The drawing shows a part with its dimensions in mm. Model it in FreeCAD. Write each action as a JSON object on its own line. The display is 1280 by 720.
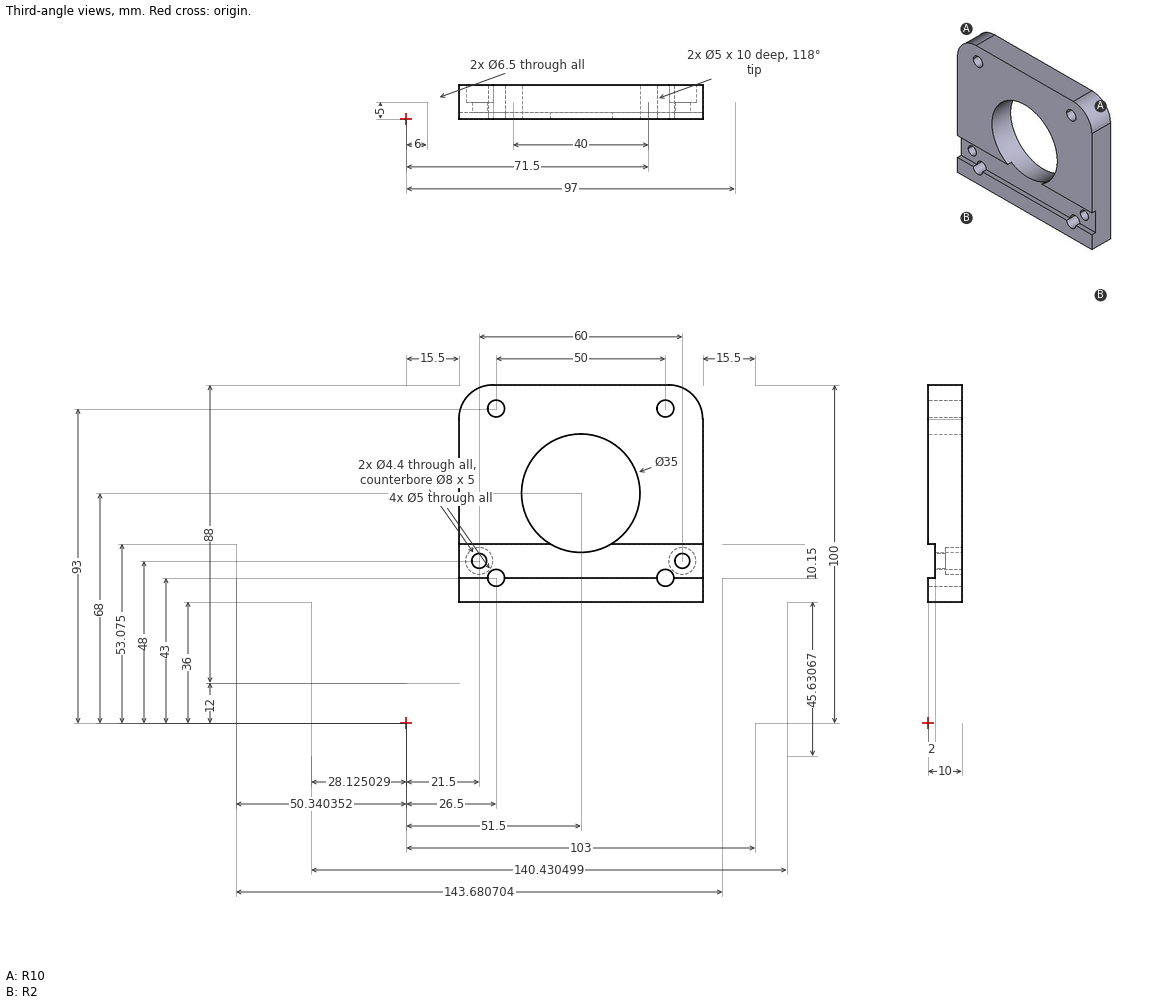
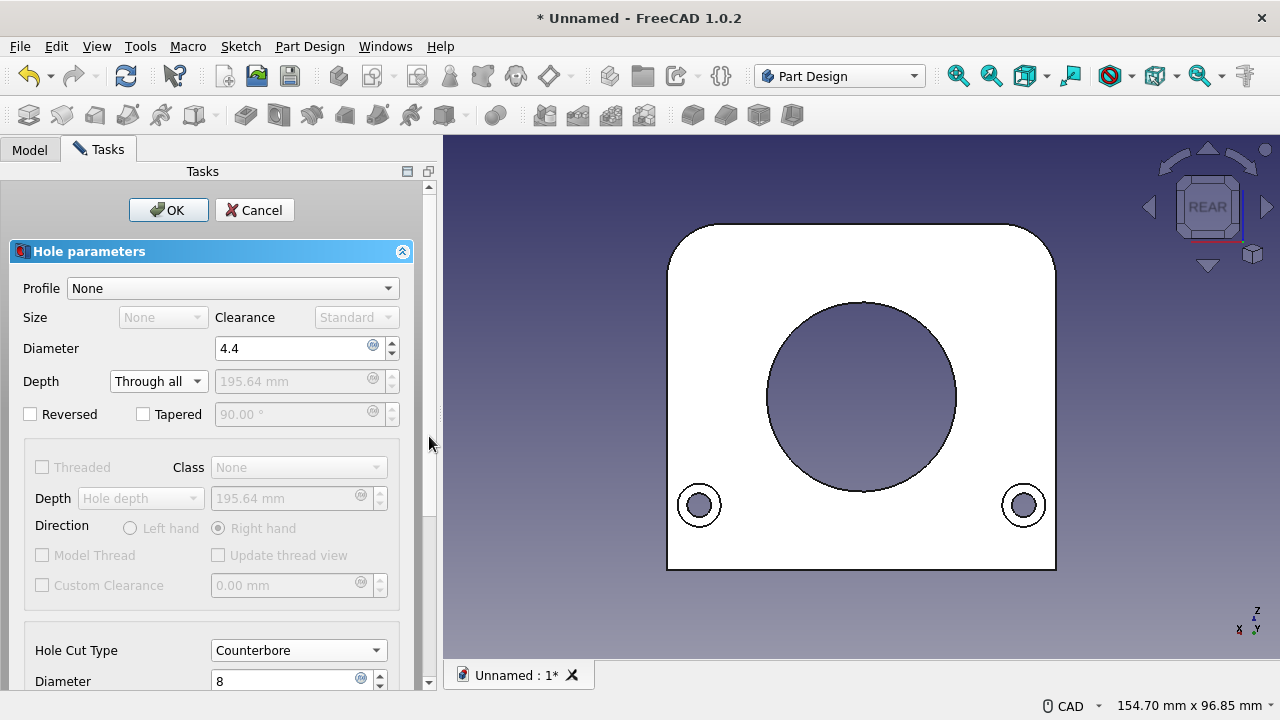
{"action": "left_click", "coordinate": [169, 210]}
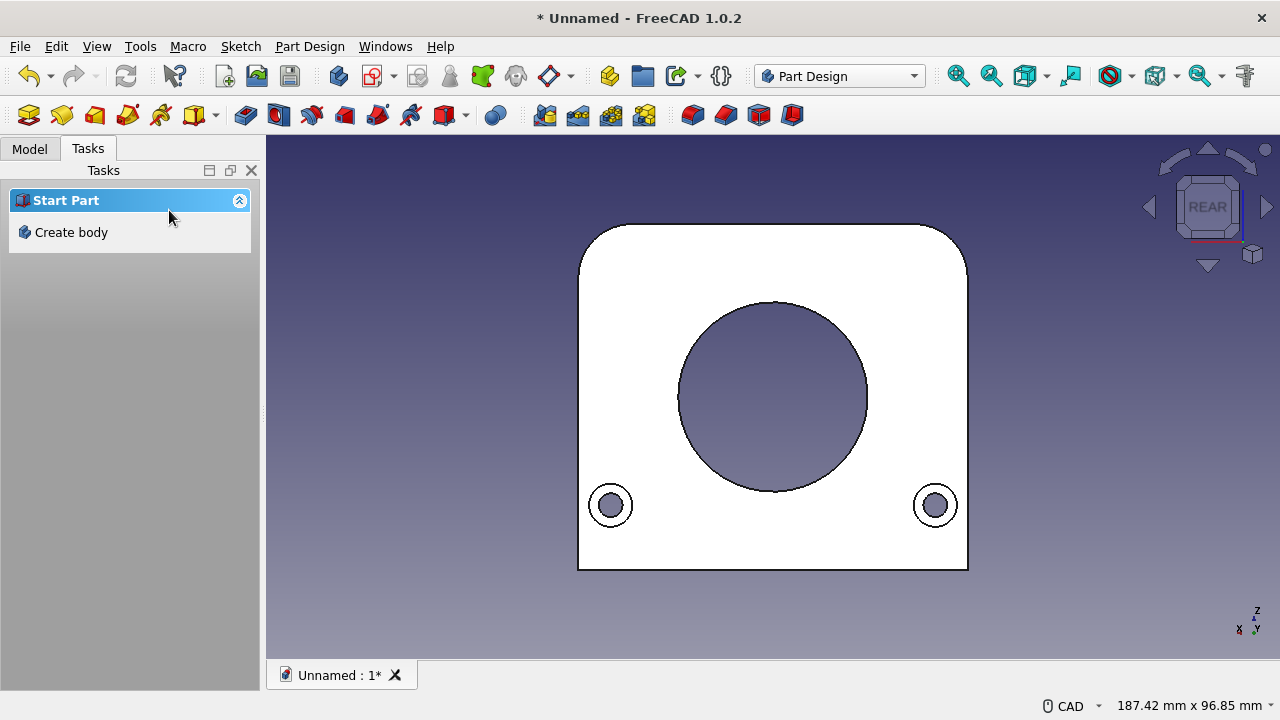
{"action": "left_click", "coordinate": [662, 297]}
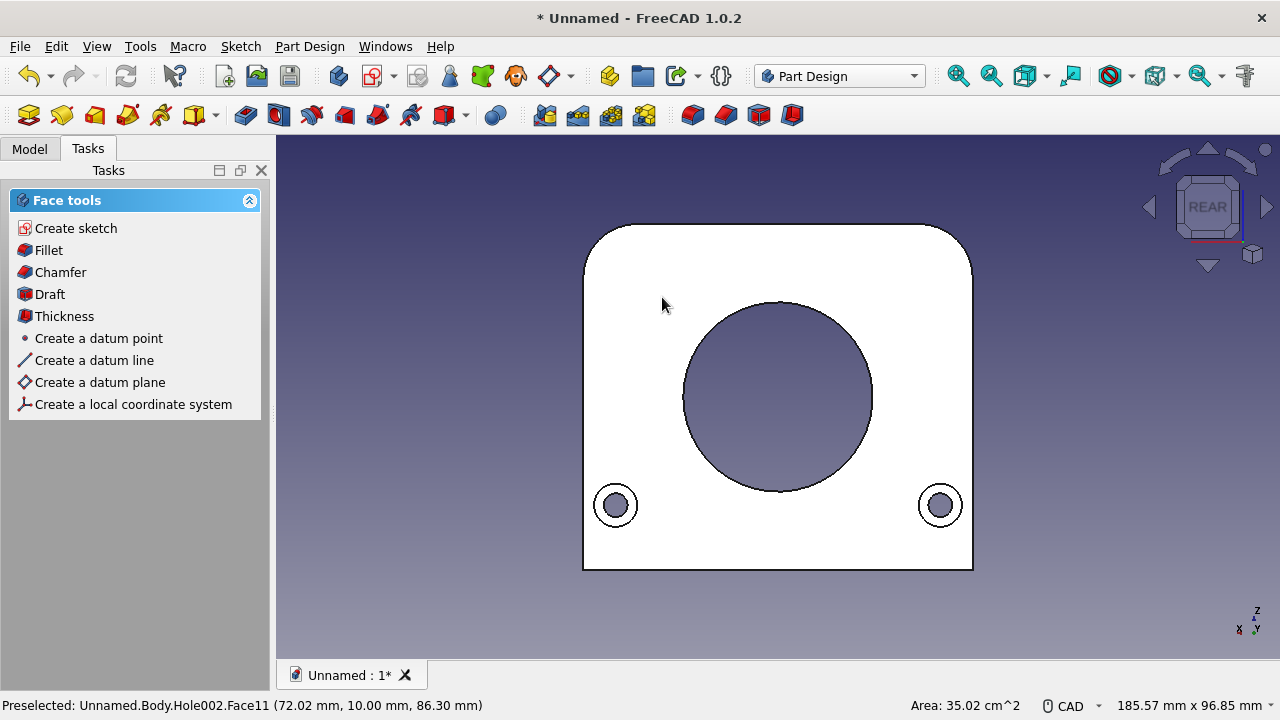
{"action": "left_click", "coordinate": [372, 76]}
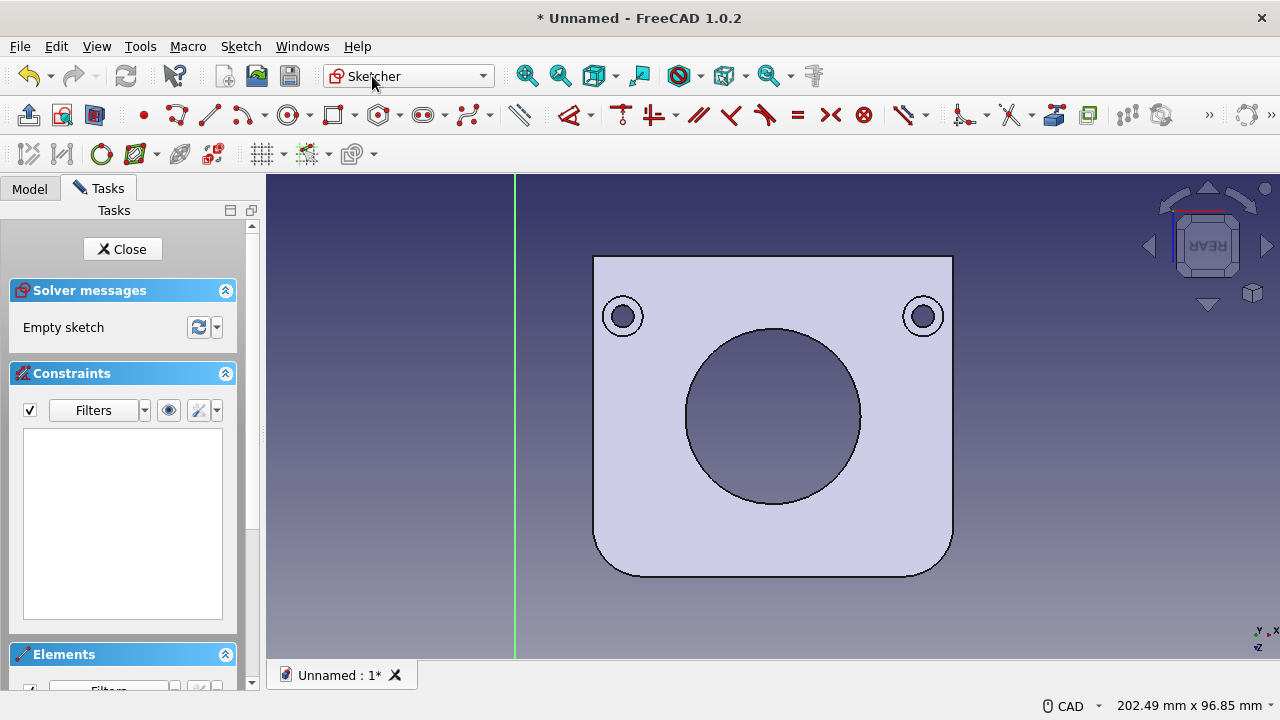
{"action": "scroll", "coordinate": [687, 623], "scroll_direction": "down", "scroll_amount": 2}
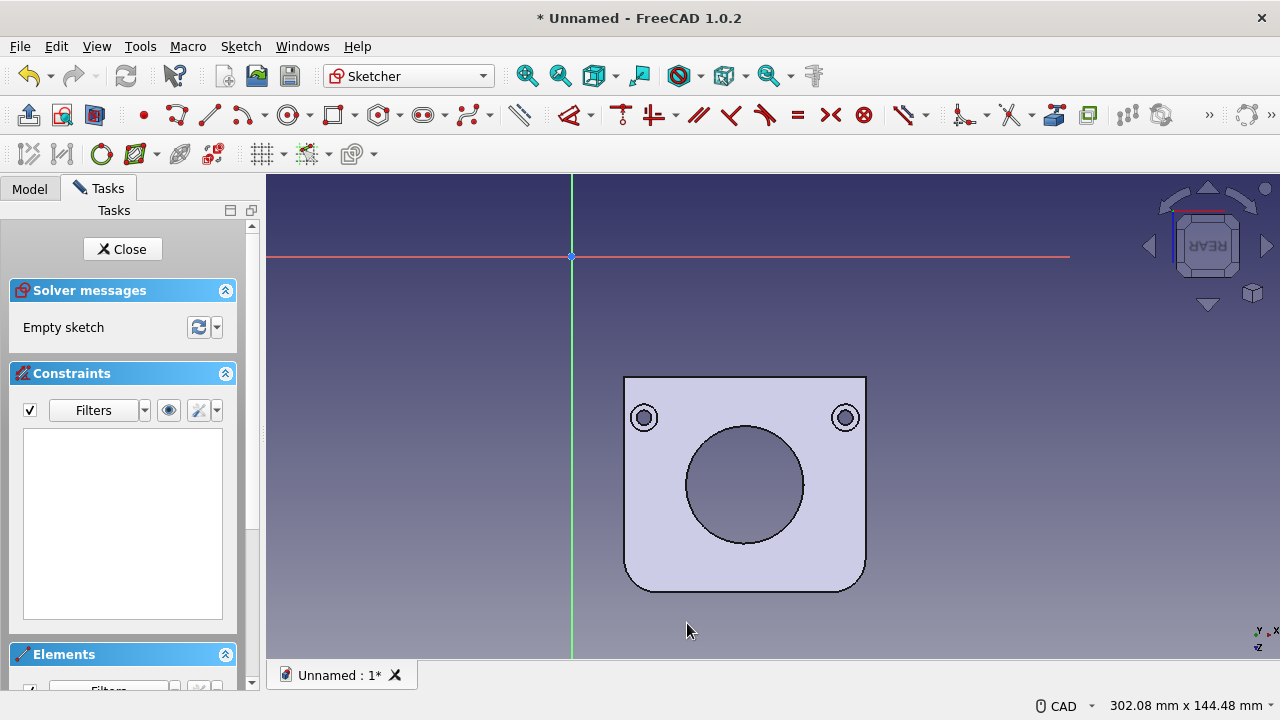
{"action": "left_click", "coordinate": [288, 116]}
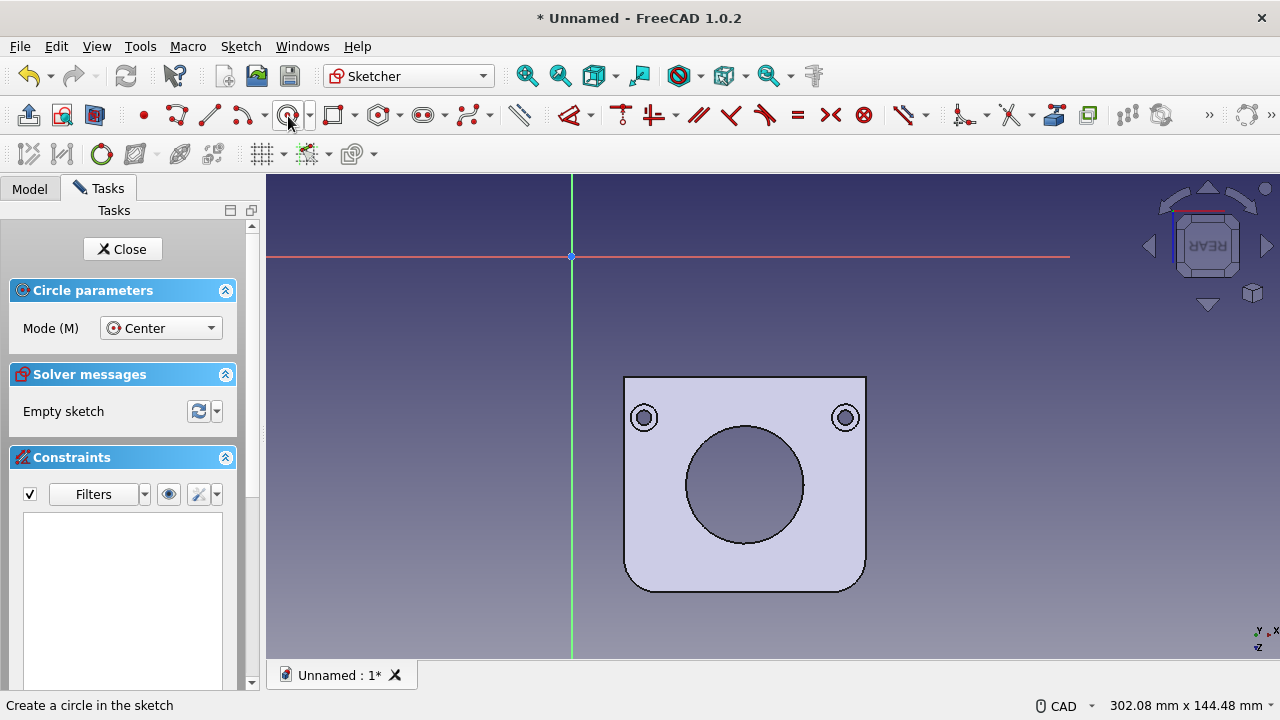
{"action": "scroll", "coordinate": [661, 401], "scroll_direction": "up", "scroll_amount": 5}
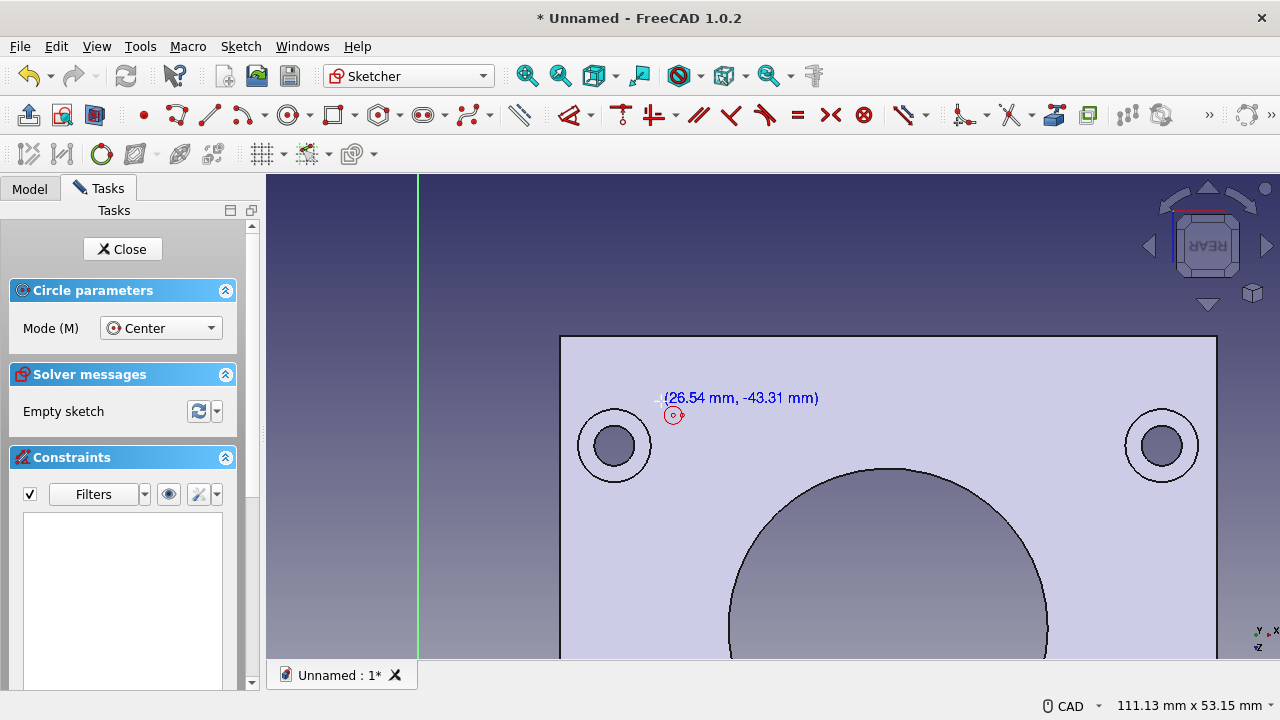
{"action": "left_click", "coordinate": [660, 400]}
{"action": "mouse_move", "coordinate": [676, 384]}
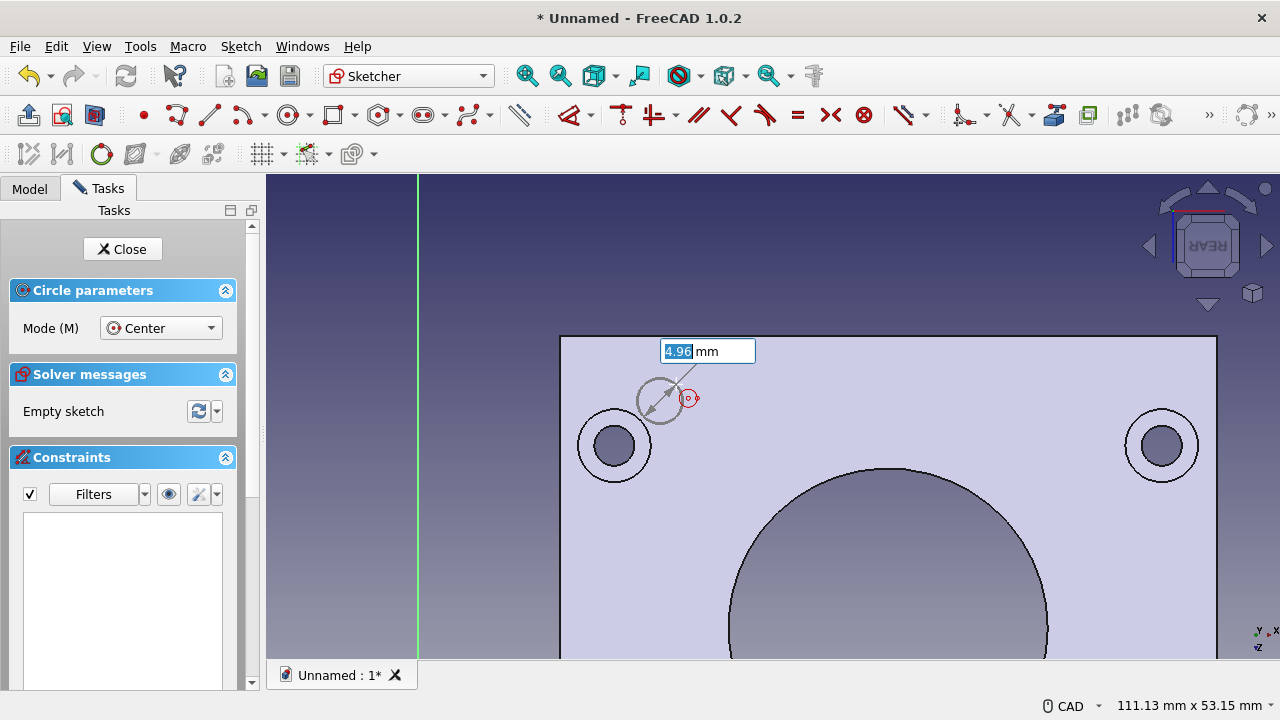
{"action": "type", "text": "5"}
{"action": "key", "text": "Return"}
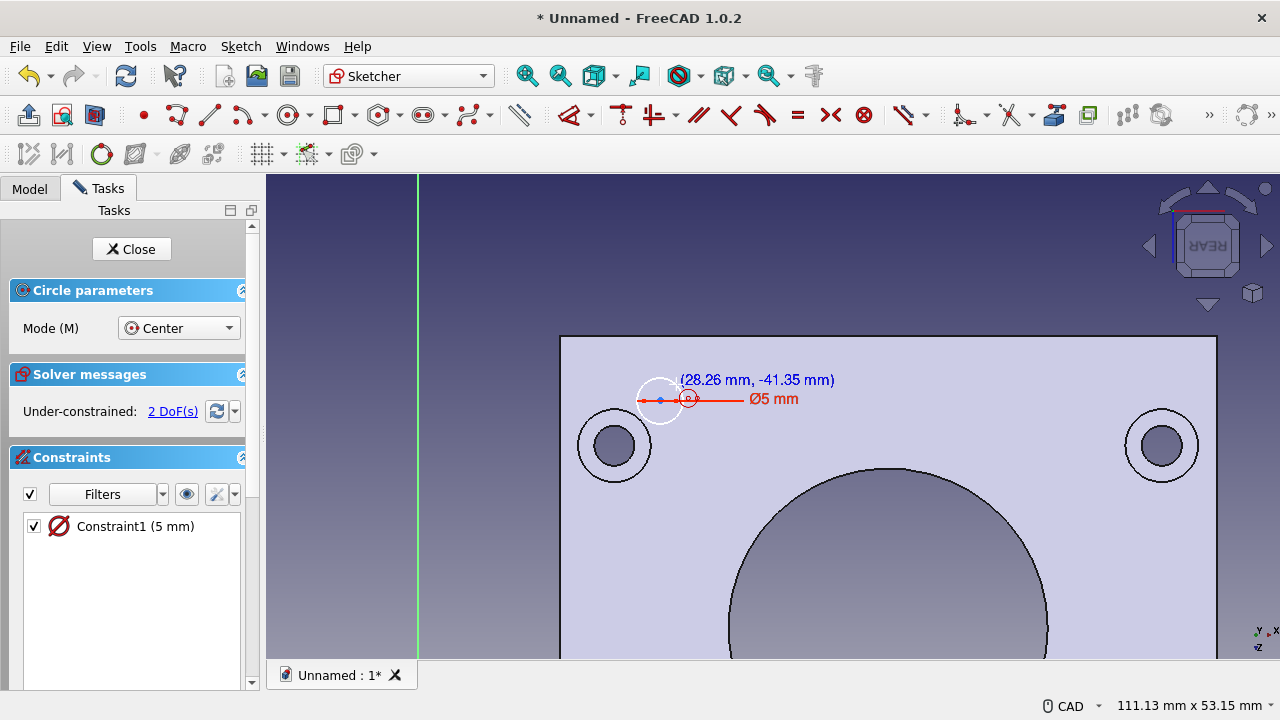
{"action": "scroll", "coordinate": [661, 401], "scroll_direction": "down", "scroll_amount": 5}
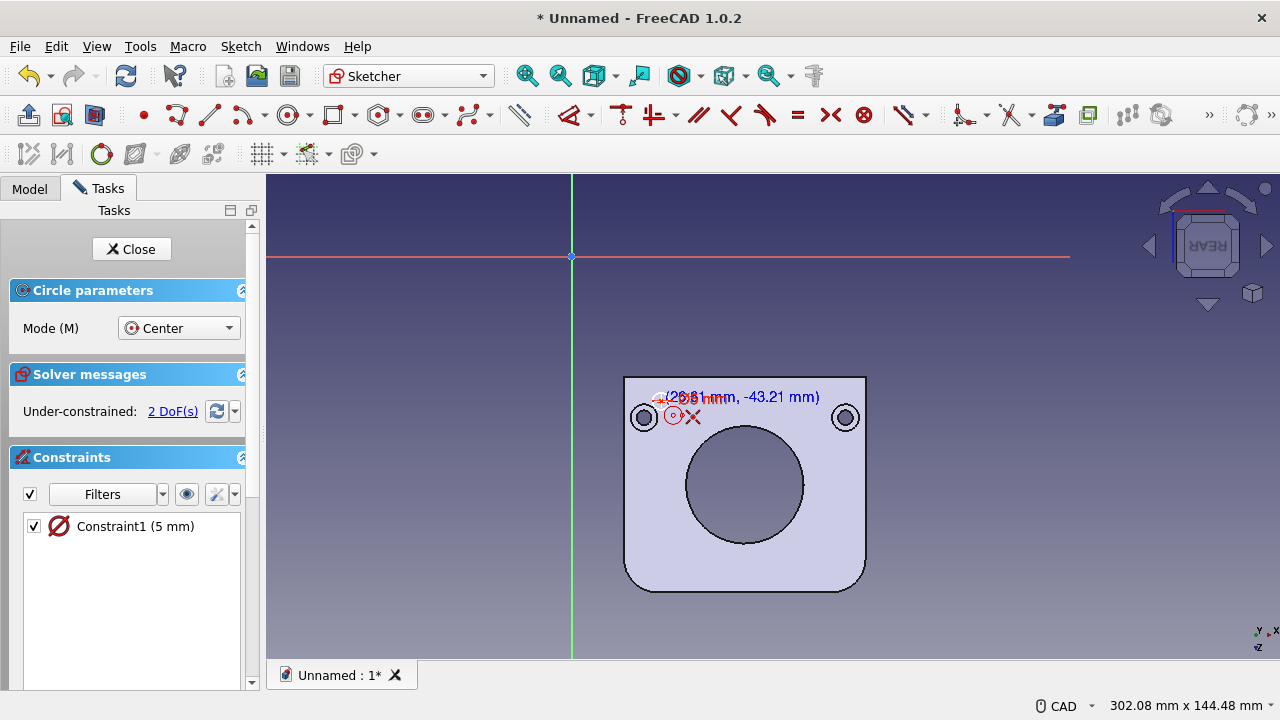
{"action": "scroll", "coordinate": [661, 569], "scroll_direction": "up", "scroll_amount": 5}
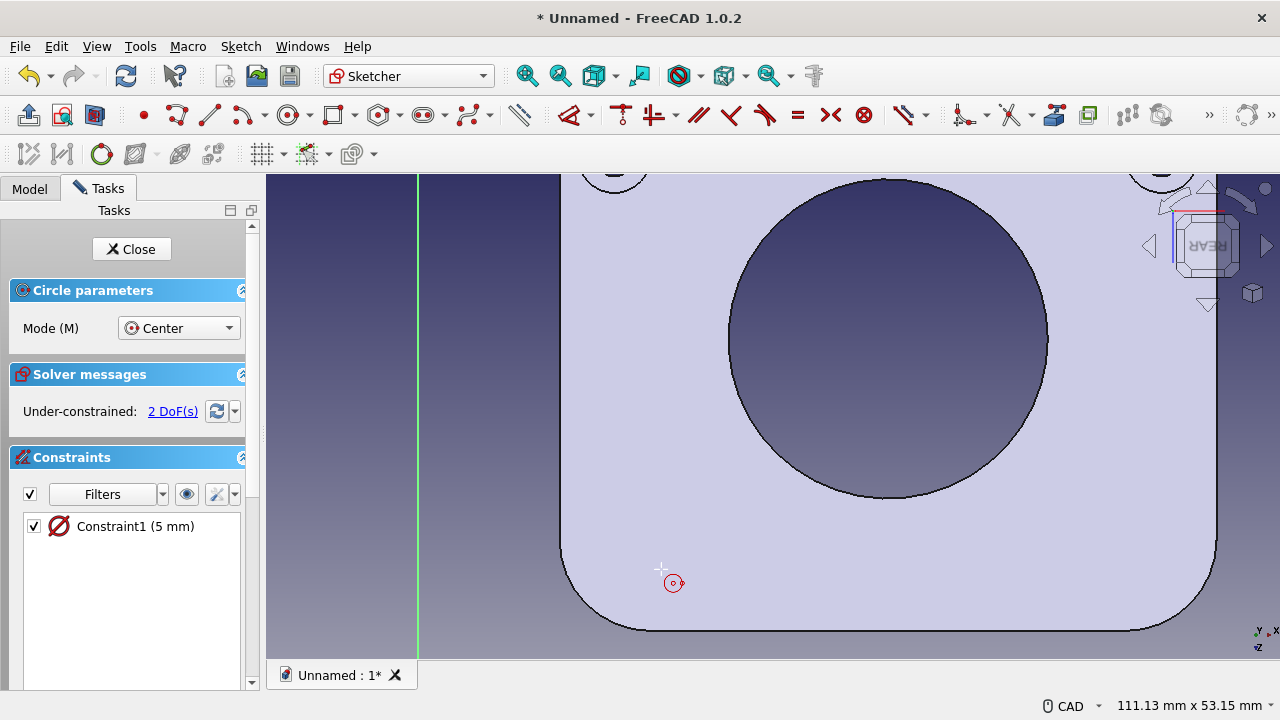
{"action": "left_click", "coordinate": [660, 567]}
{"action": "mouse_move", "coordinate": [676, 551]}